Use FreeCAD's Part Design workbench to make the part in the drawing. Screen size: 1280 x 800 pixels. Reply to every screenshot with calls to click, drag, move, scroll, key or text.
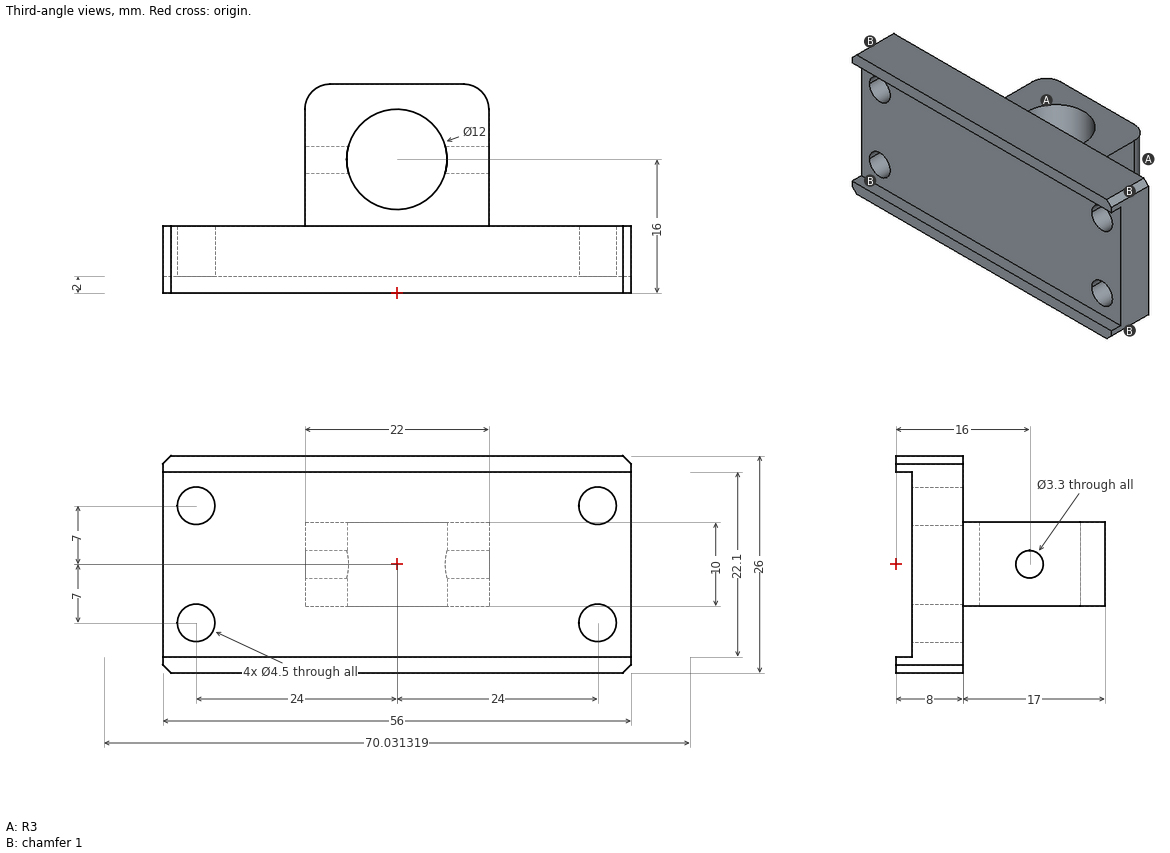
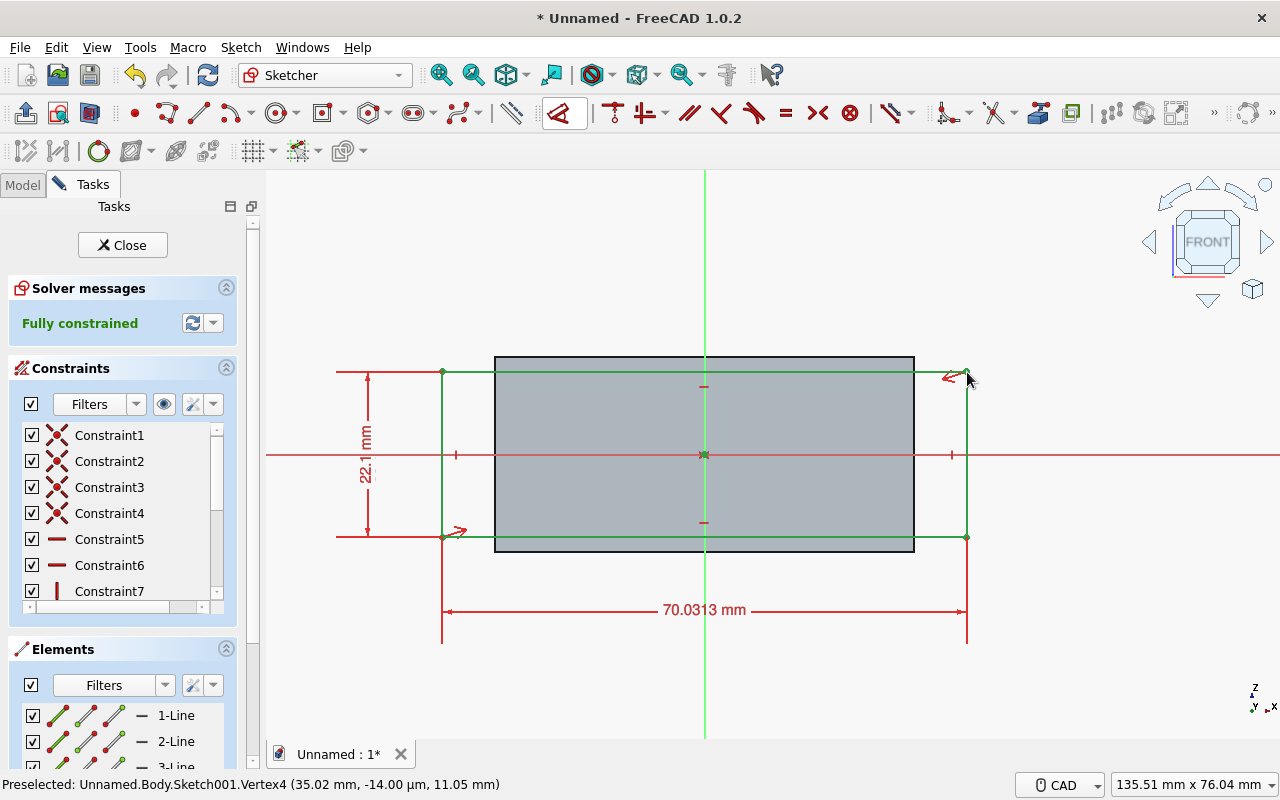
click(123, 245)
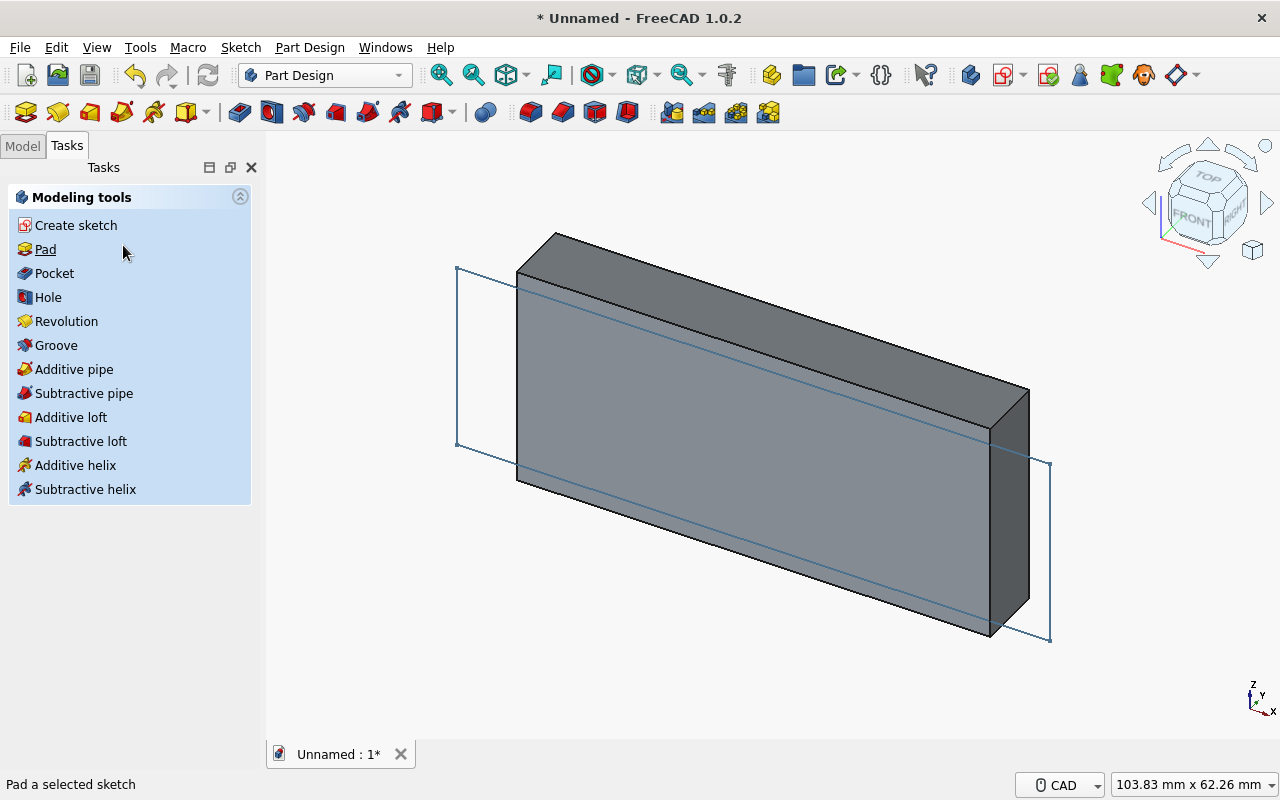
click(240, 112)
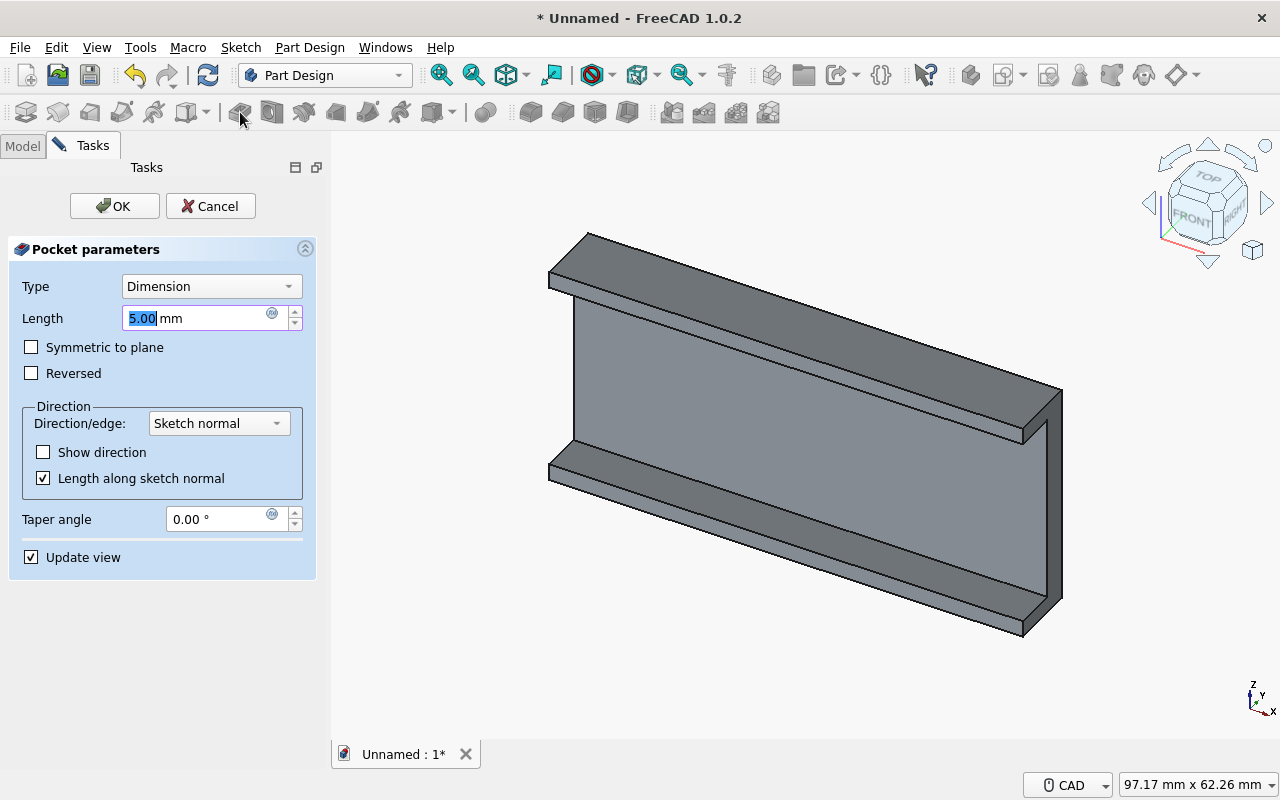
text(2)
key(Tab)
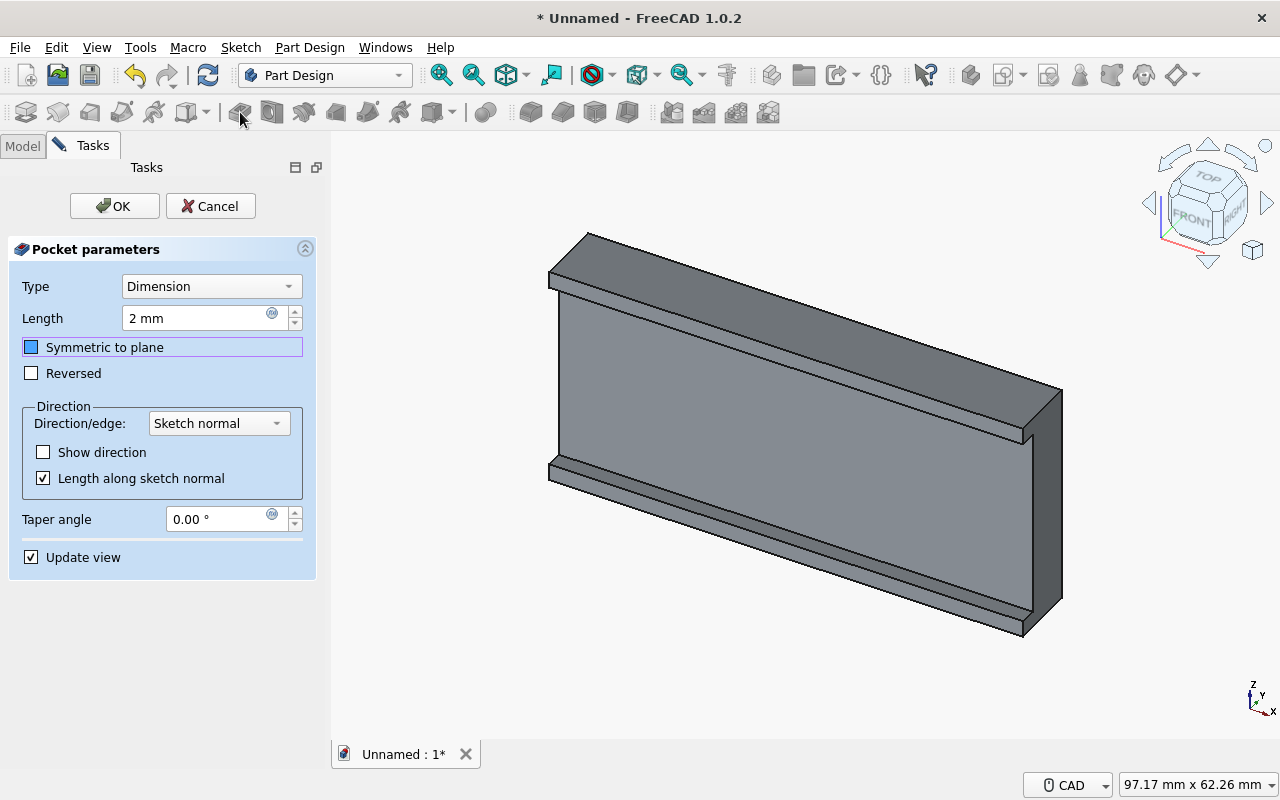
click(115, 206)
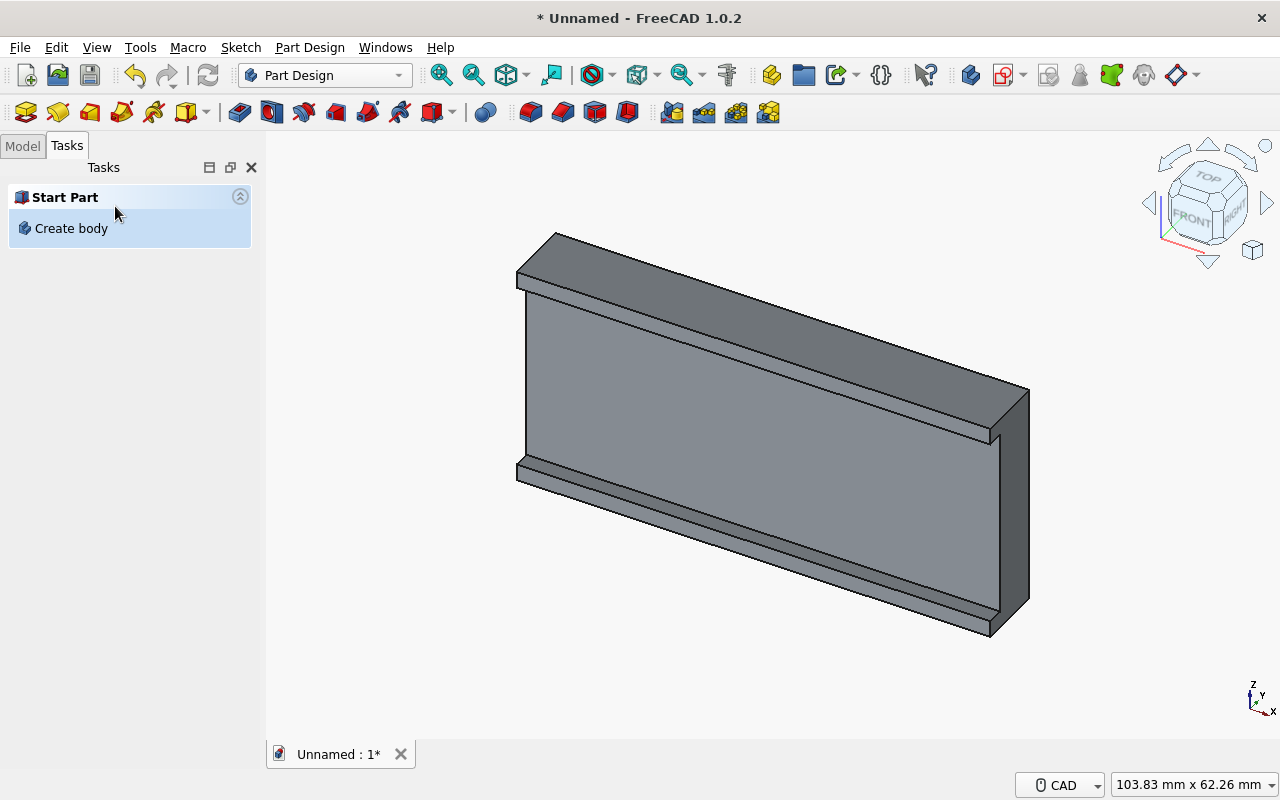
key(4)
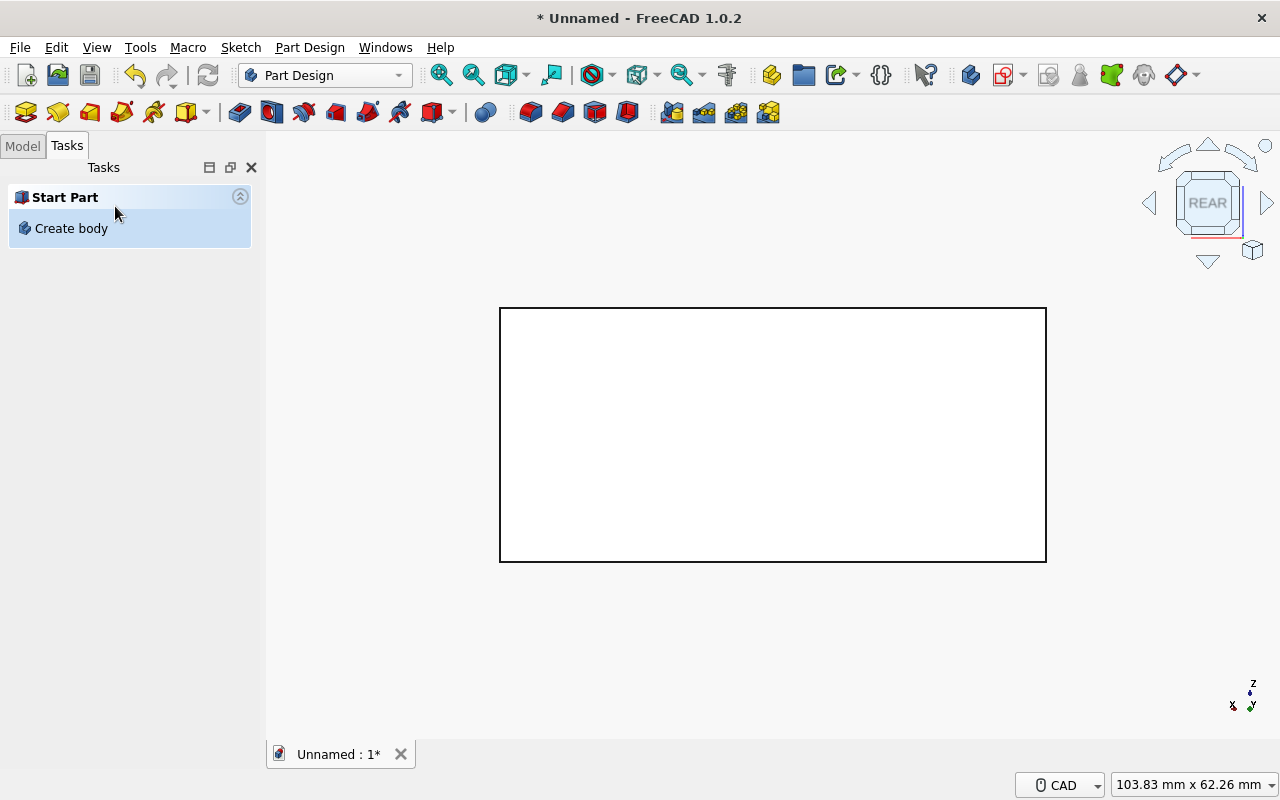
click(695, 434)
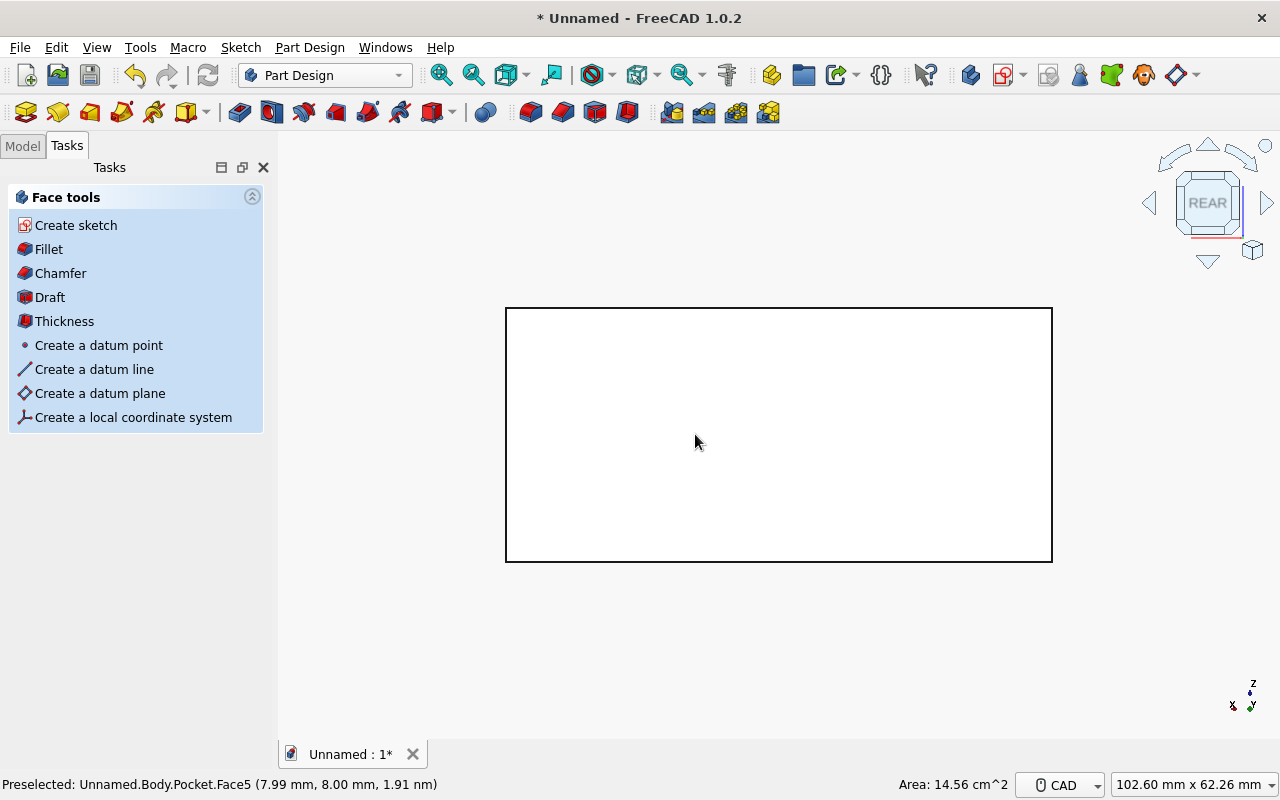
click(1004, 76)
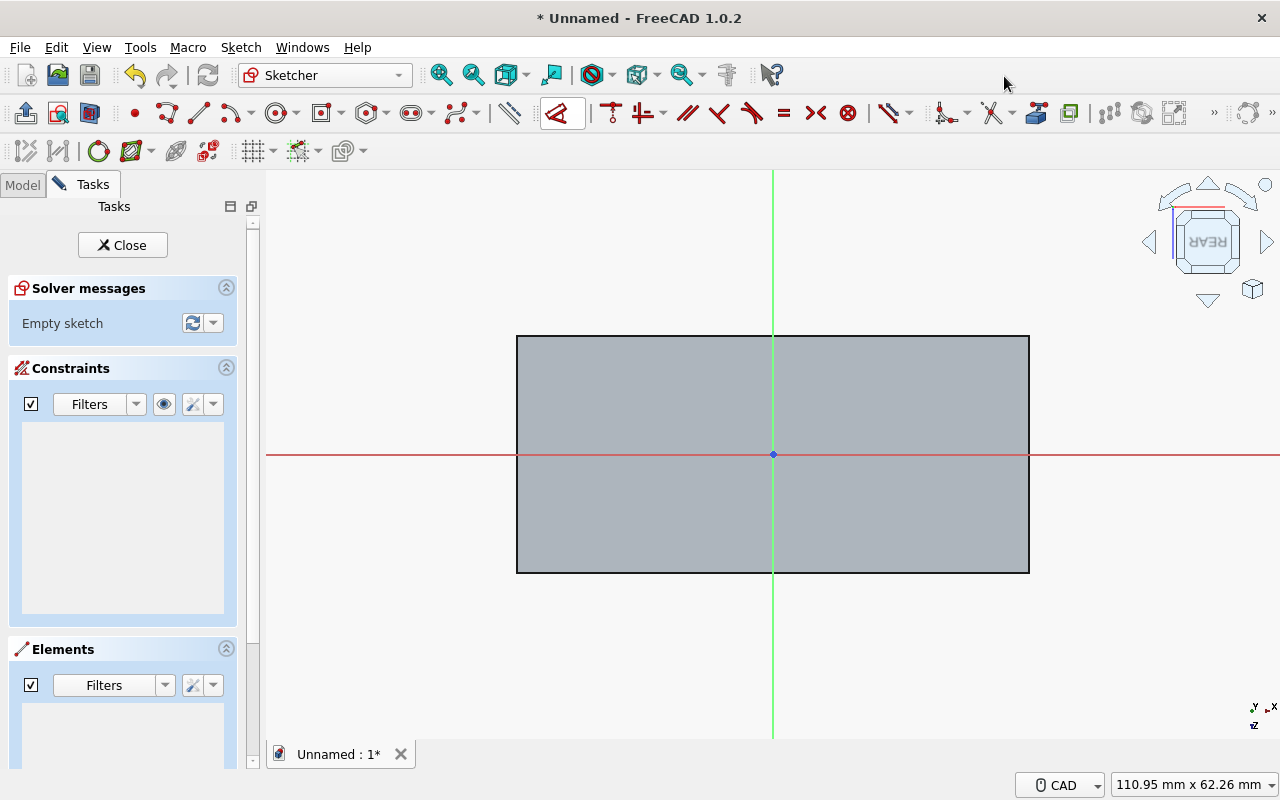
scroll(813, 454, up, 5)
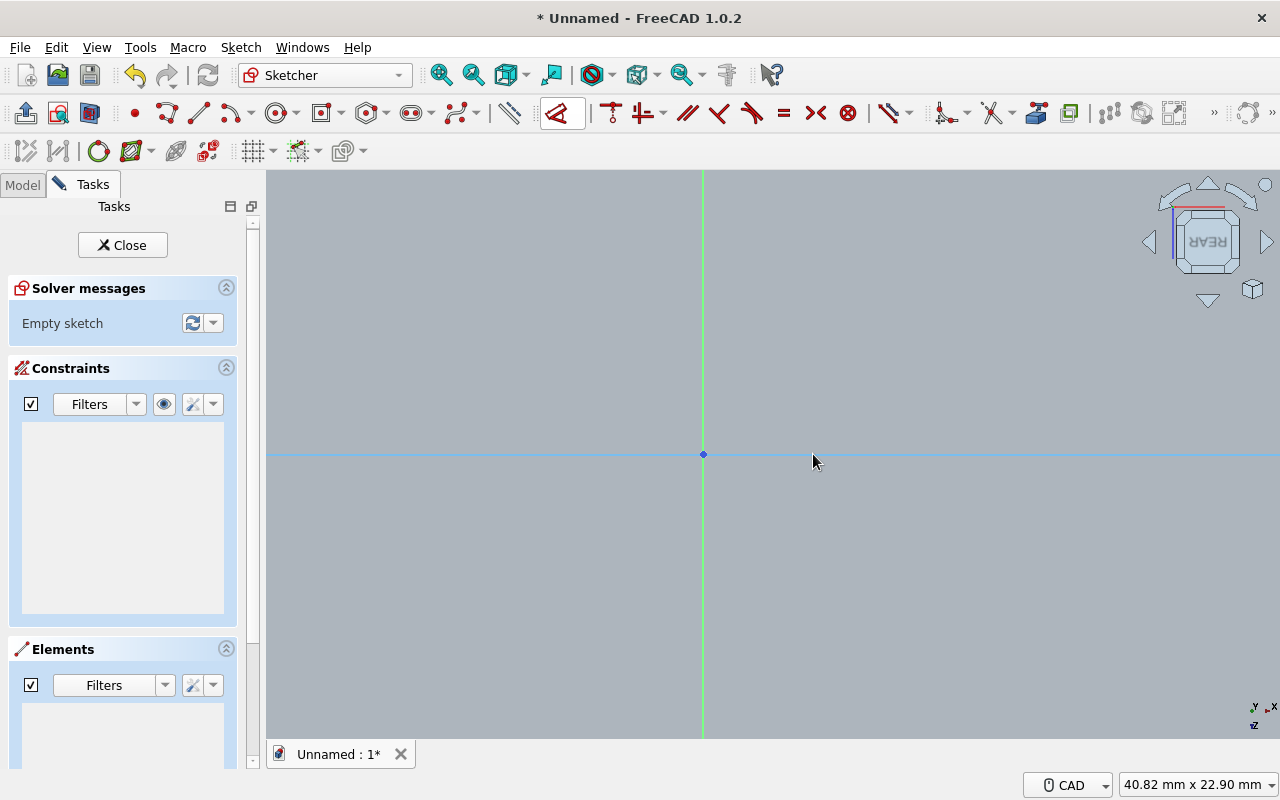
click(322, 114)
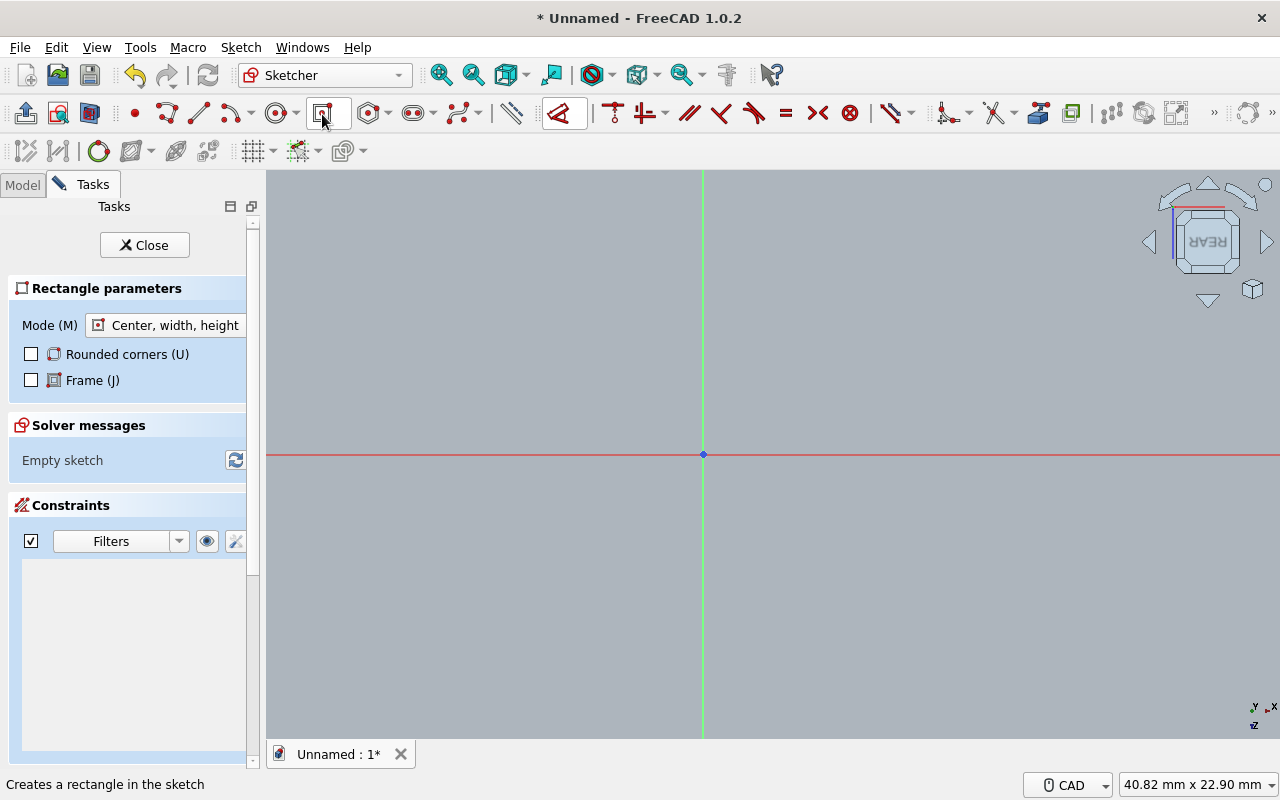
click(703, 454)
move(977, 330)